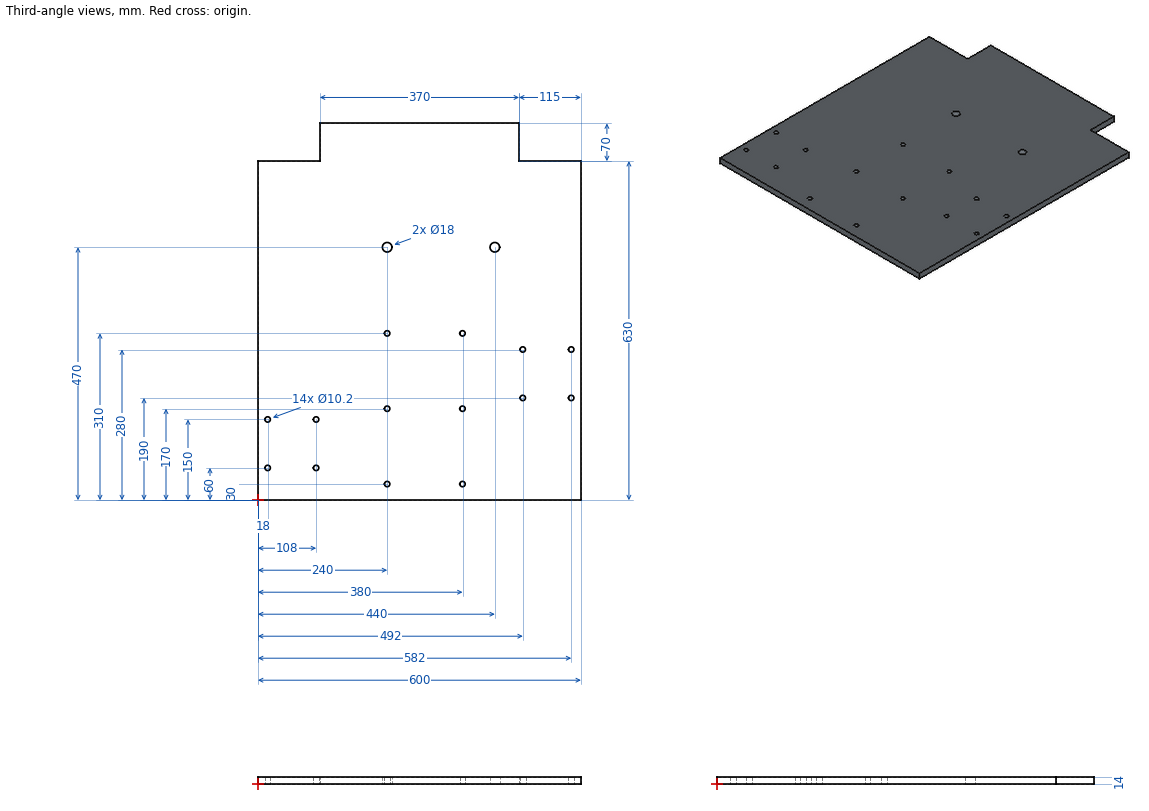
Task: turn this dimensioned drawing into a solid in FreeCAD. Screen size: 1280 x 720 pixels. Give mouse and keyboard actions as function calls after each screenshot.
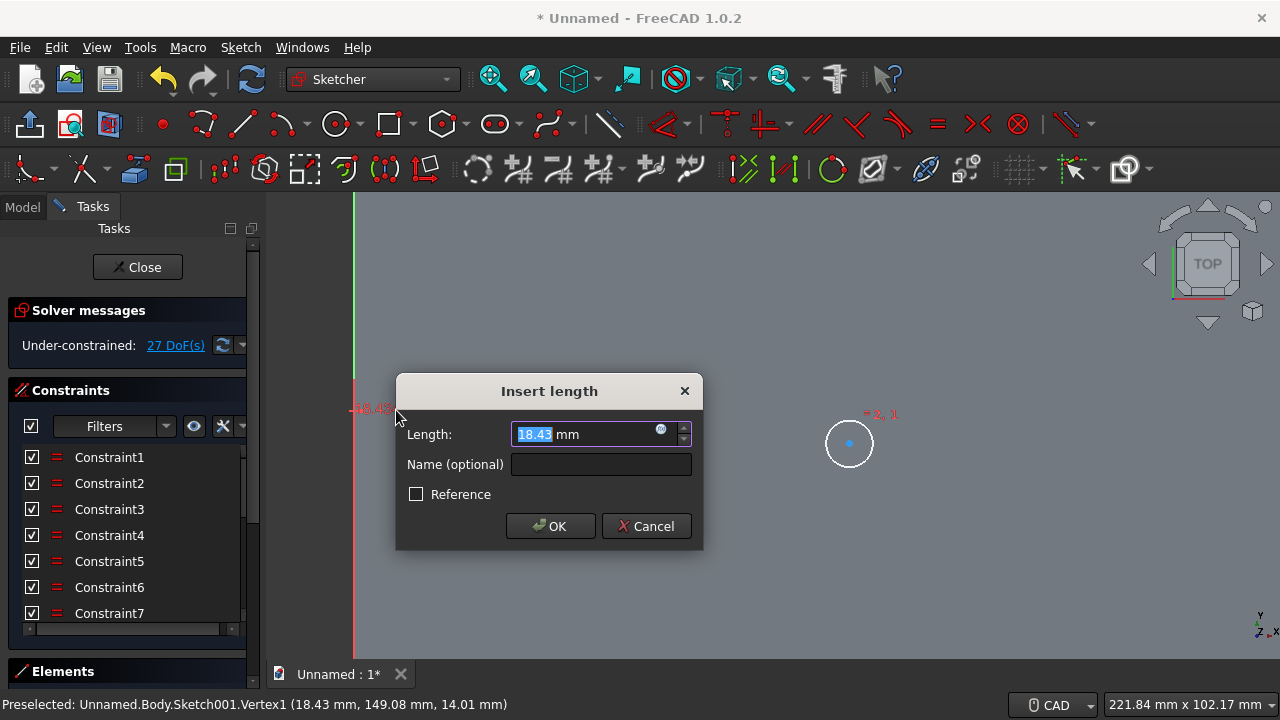
text(18)
key(Return)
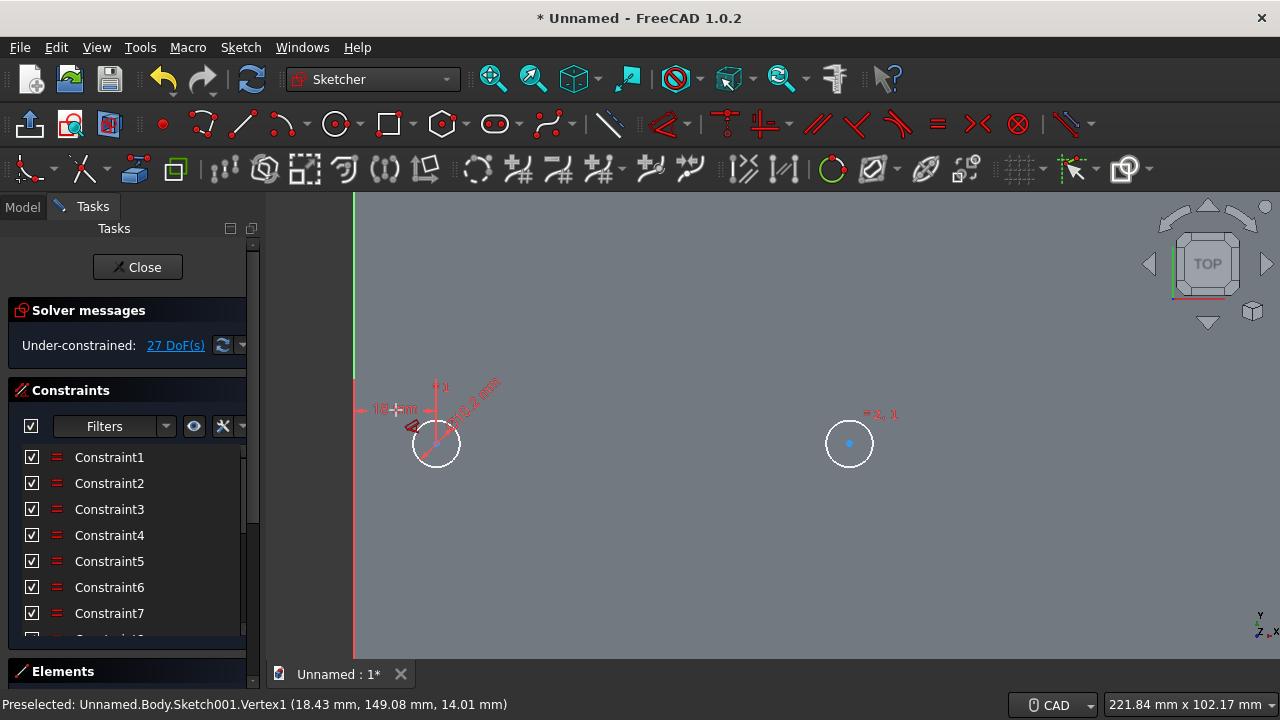
scroll(454, 431, down, 8)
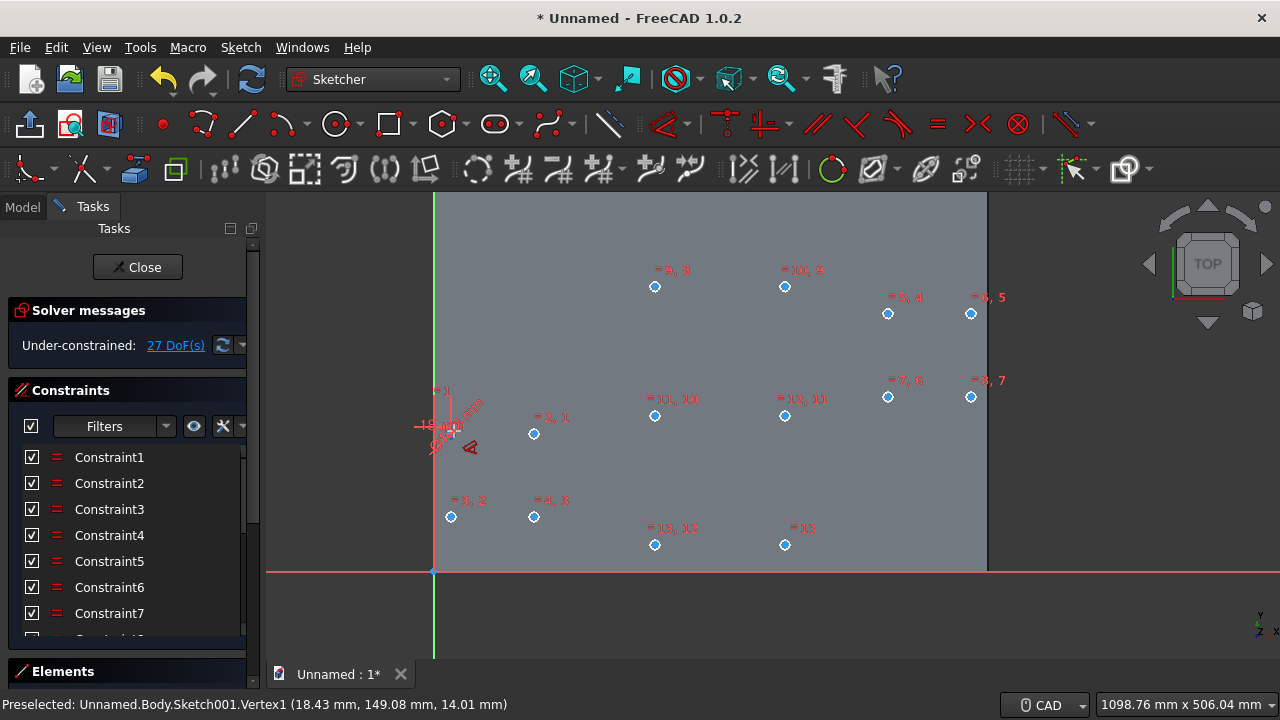
scroll(451, 517, up, 5)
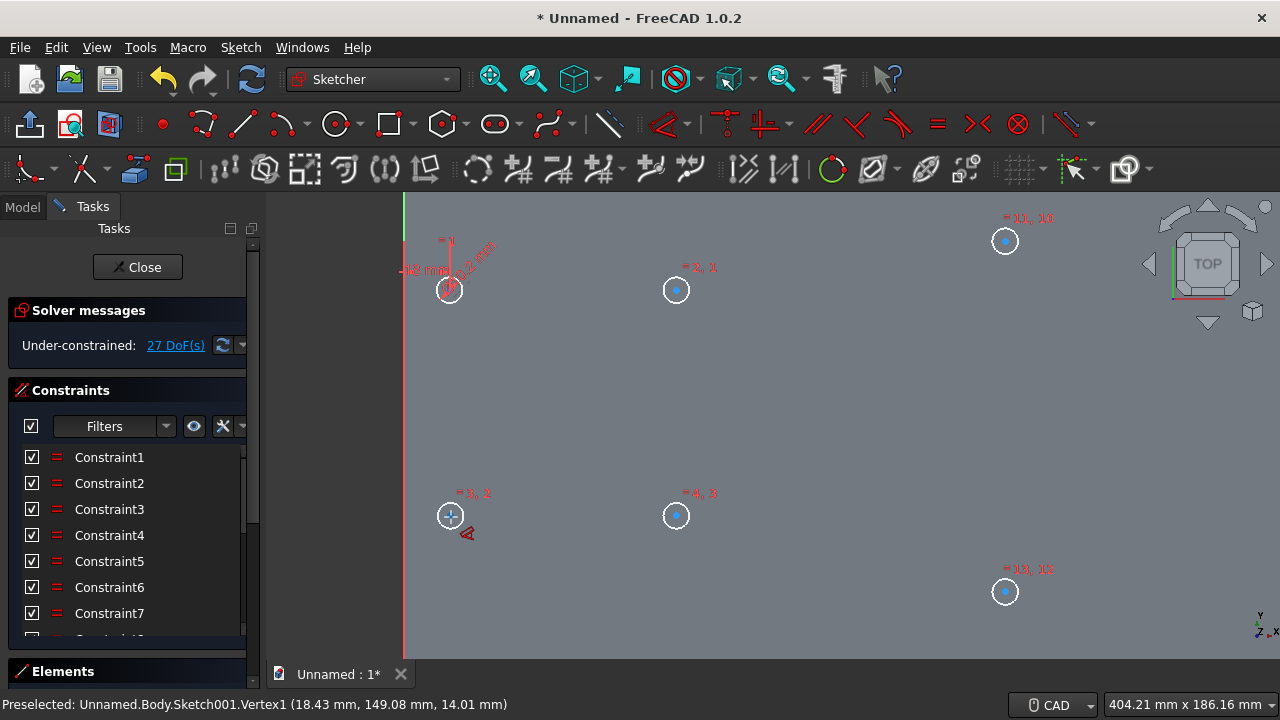
click(451, 516)
click(428, 482)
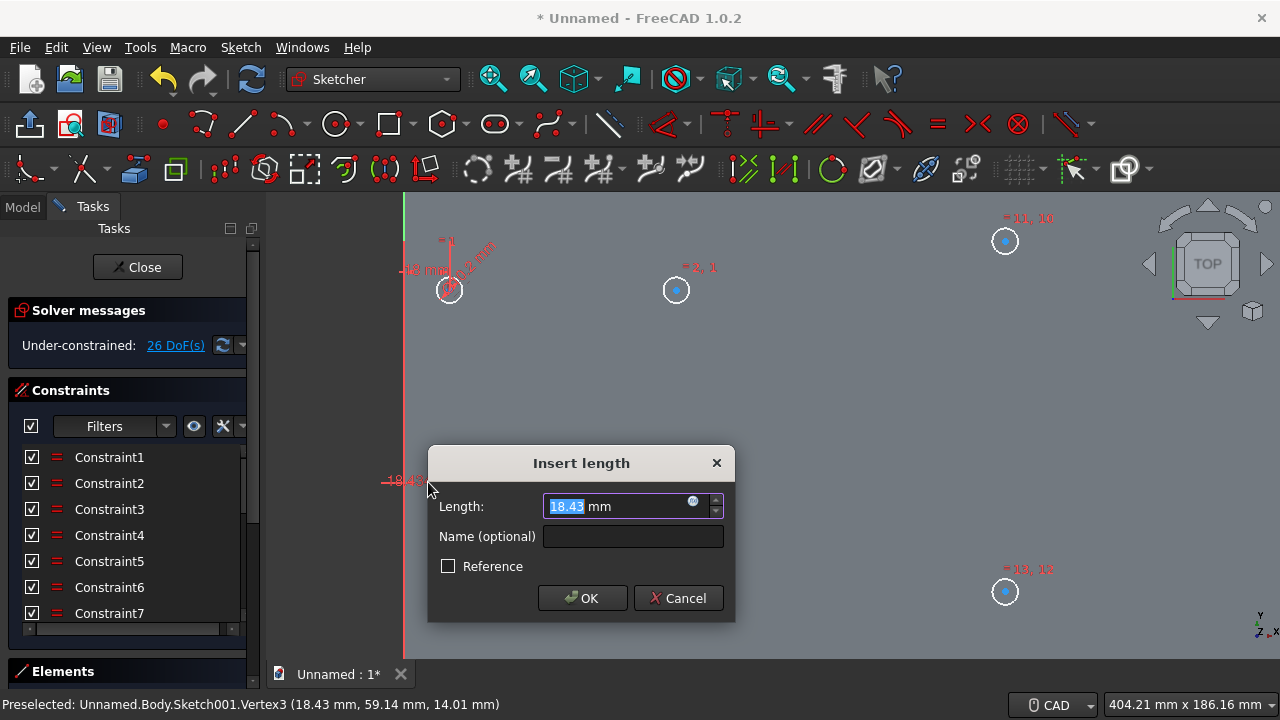
text(18)
key(Return)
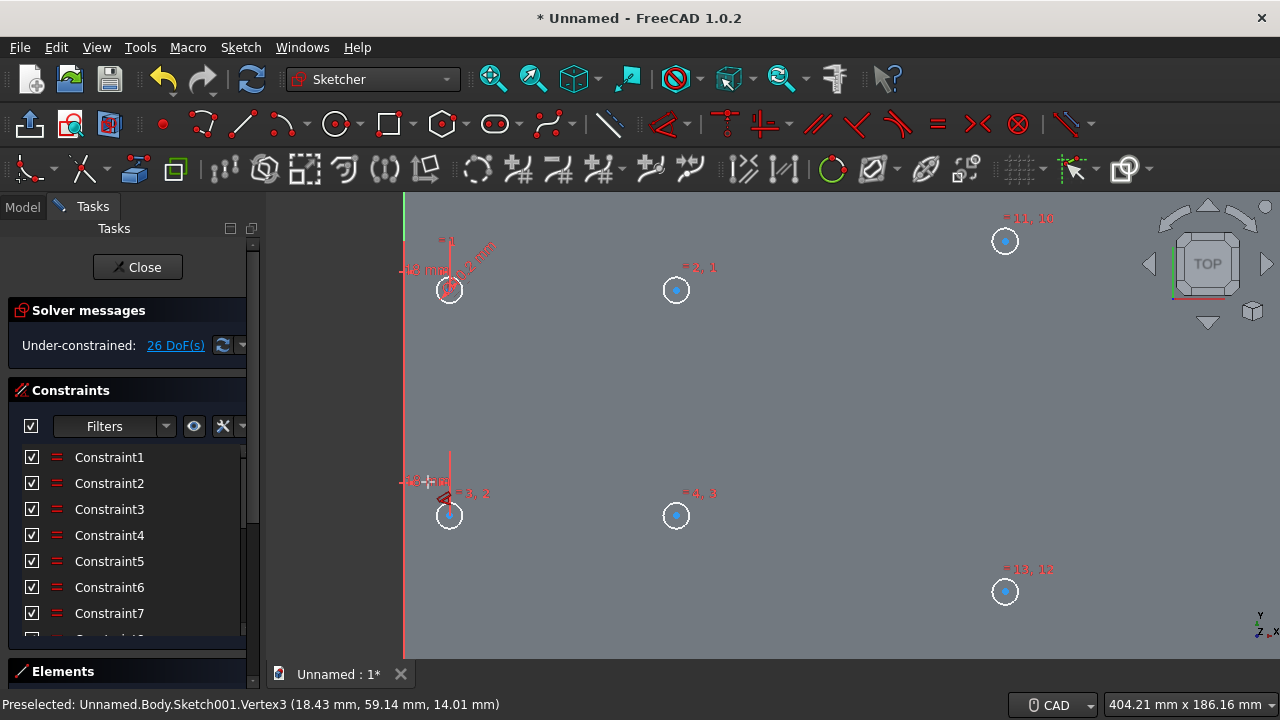
click(450, 516)
click(370, 573)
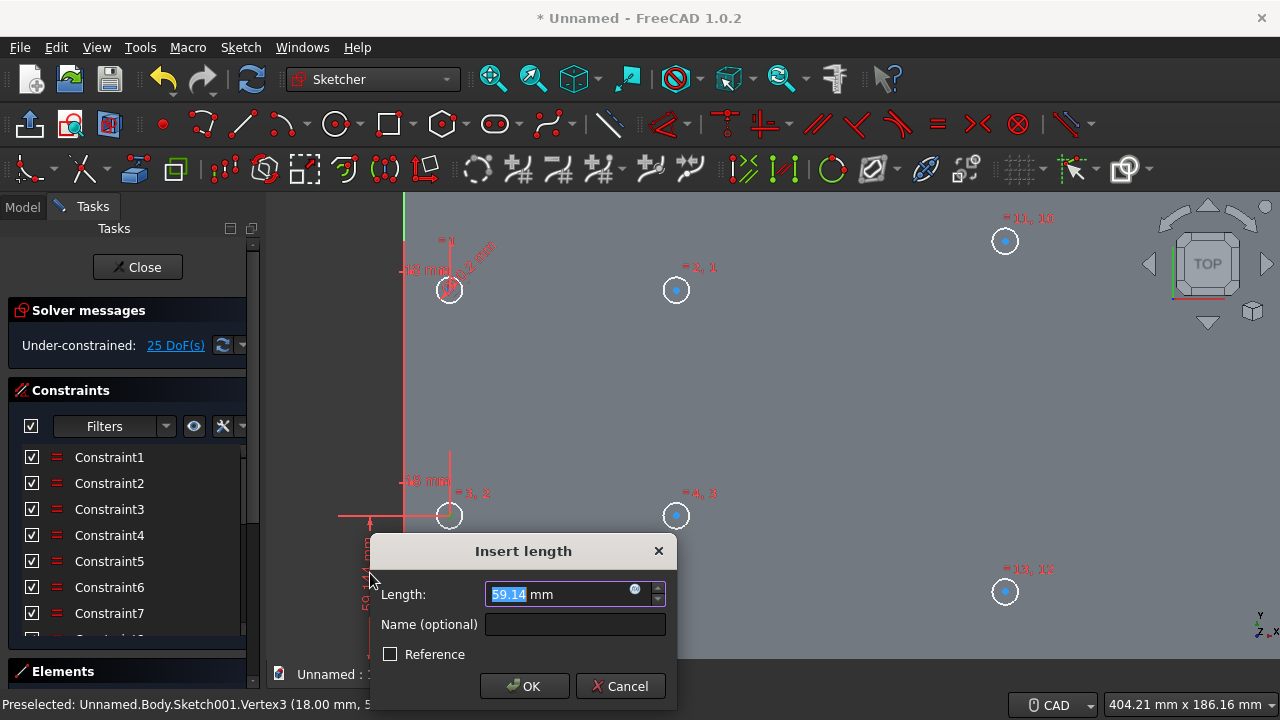
text(60)
key(Return)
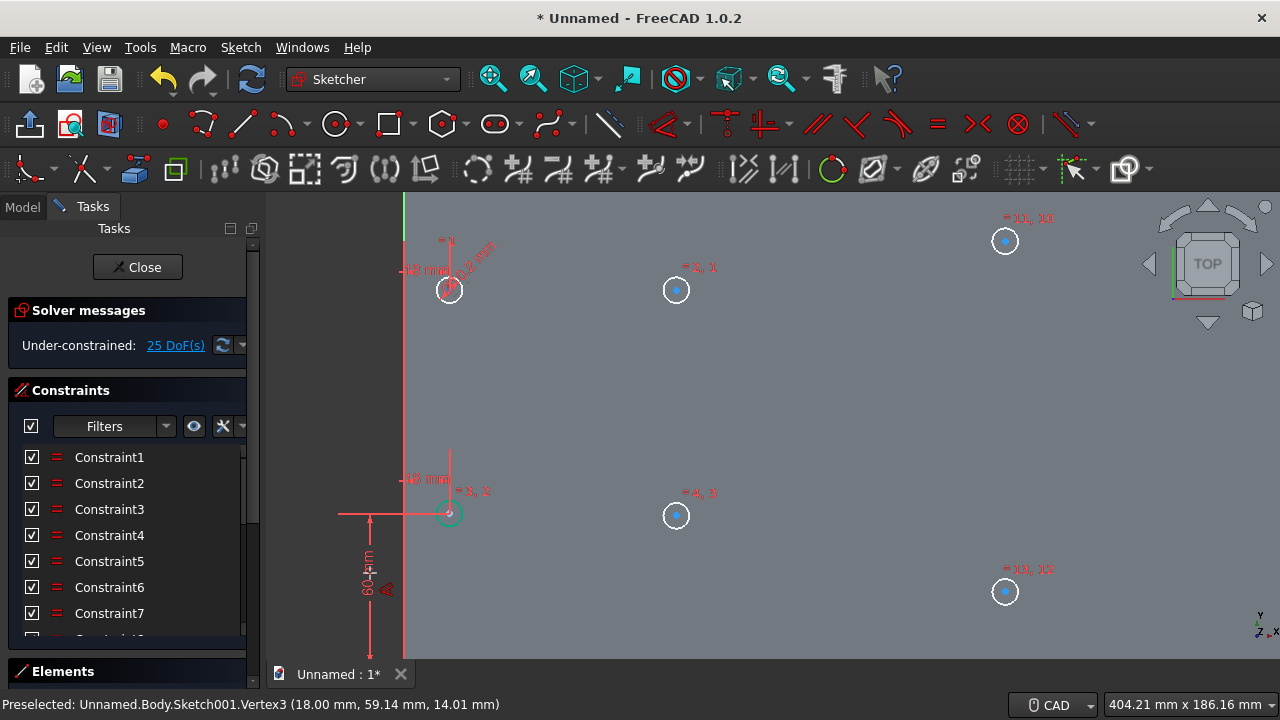
click(676, 516)
click(370, 547)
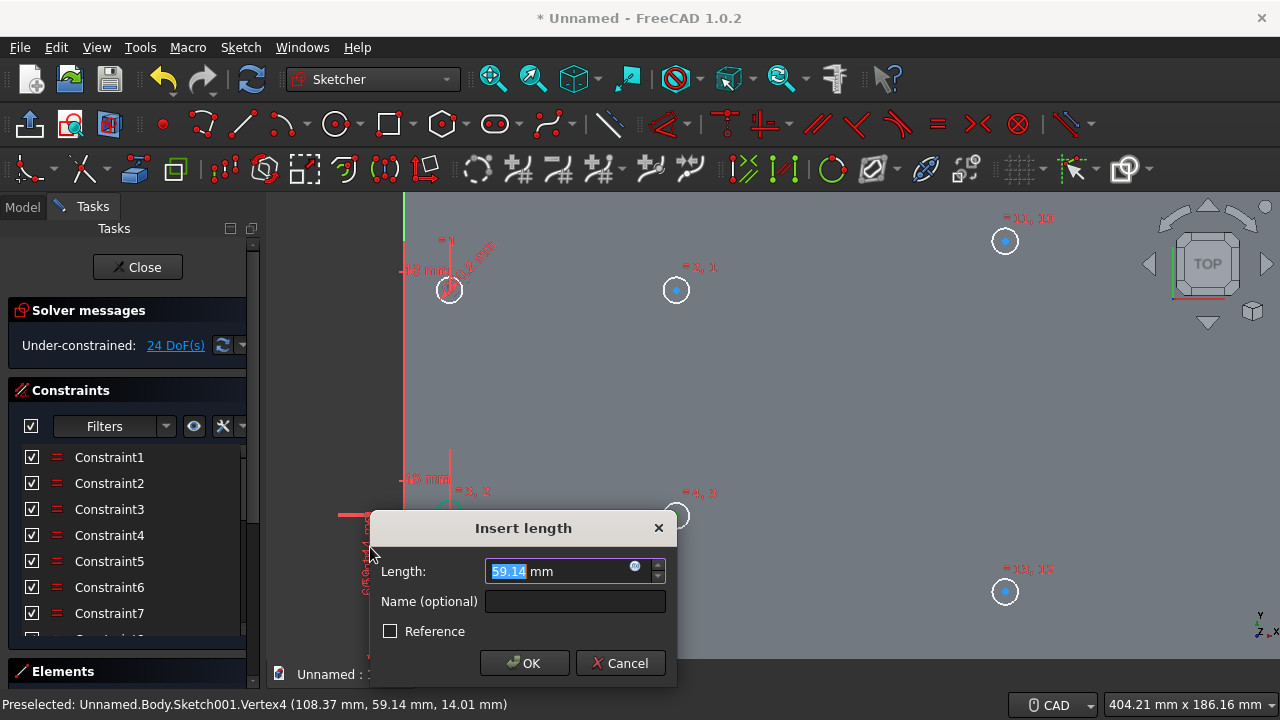
text(60)
key(Return)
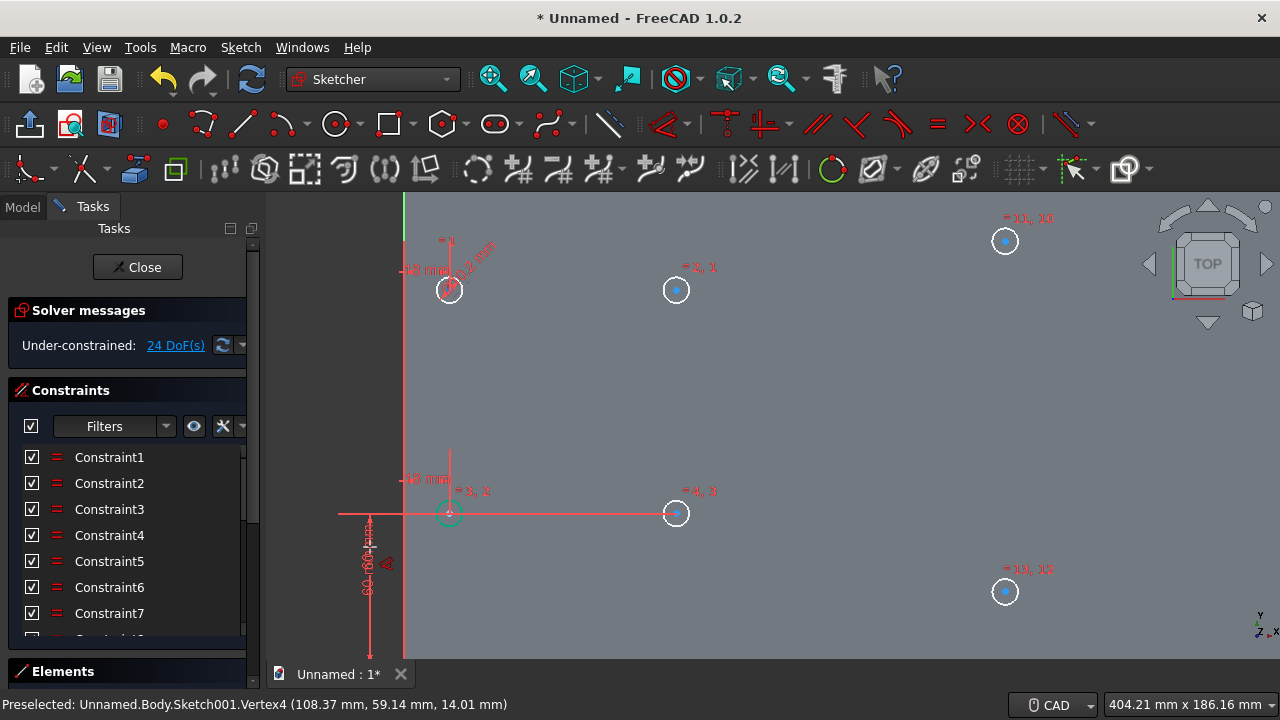
click(1005, 592)
click(370, 611)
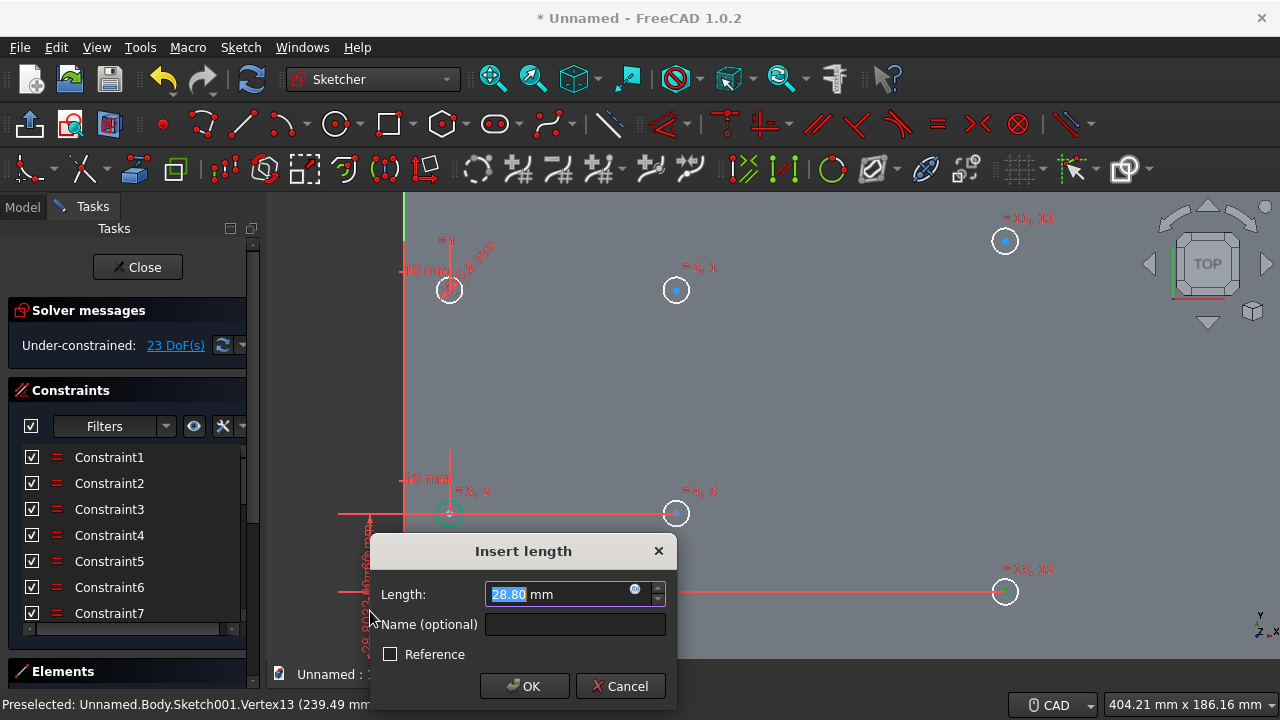
text(30)
key(Return)